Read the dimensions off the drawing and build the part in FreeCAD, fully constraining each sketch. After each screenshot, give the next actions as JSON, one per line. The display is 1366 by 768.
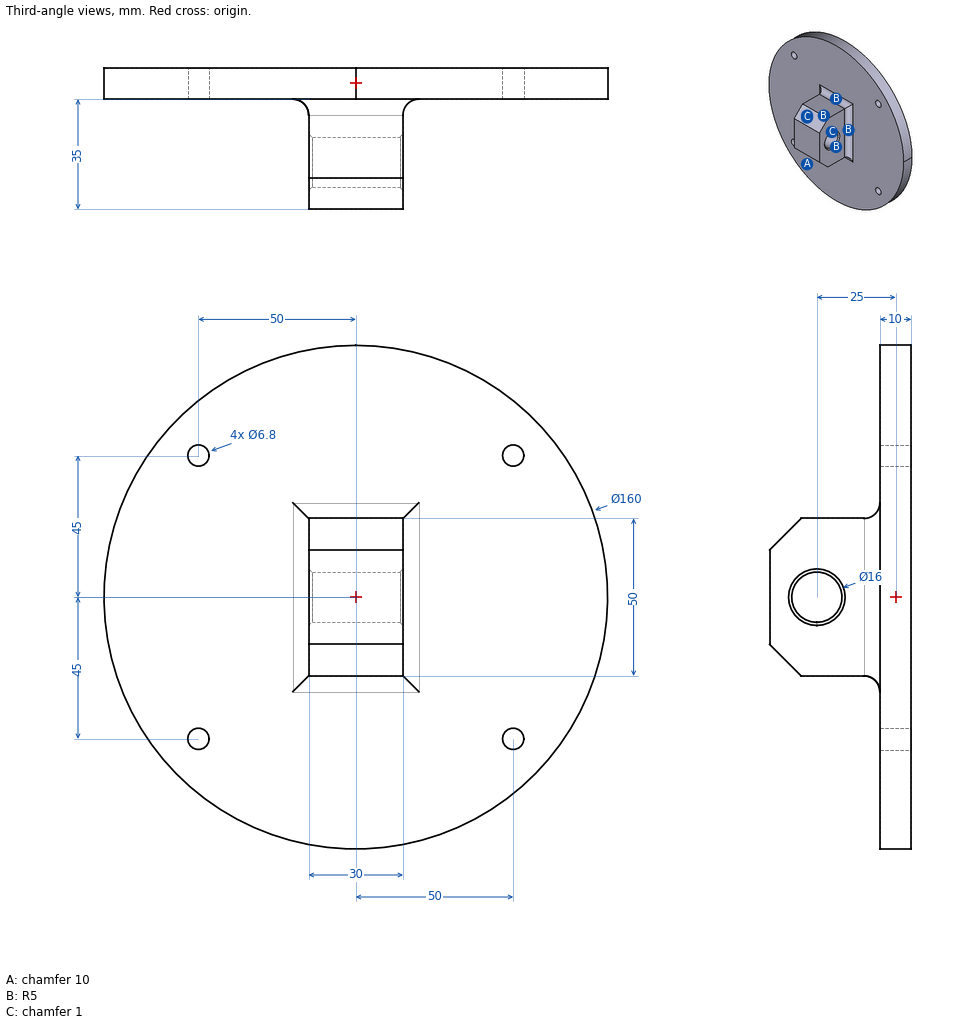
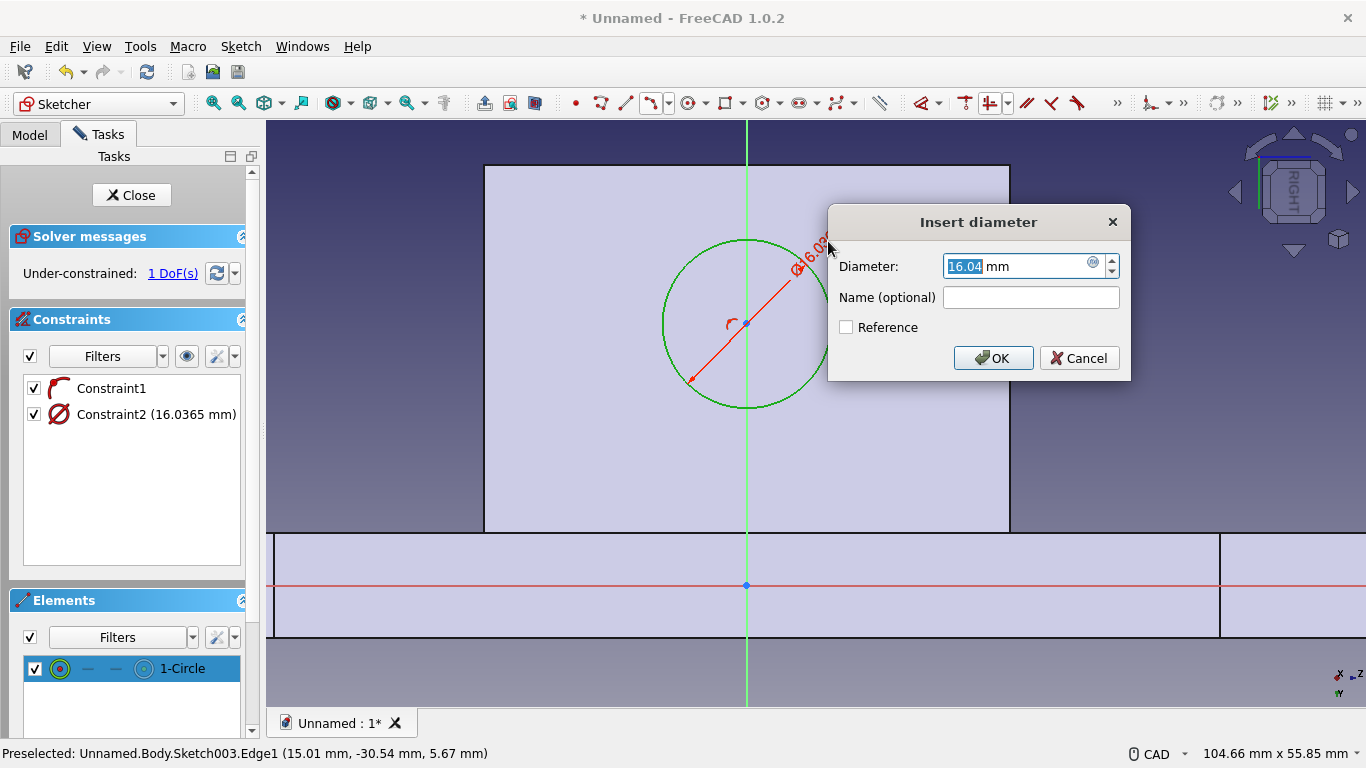
{"action": "type", "text": "16"}
{"action": "key", "text": "Return"}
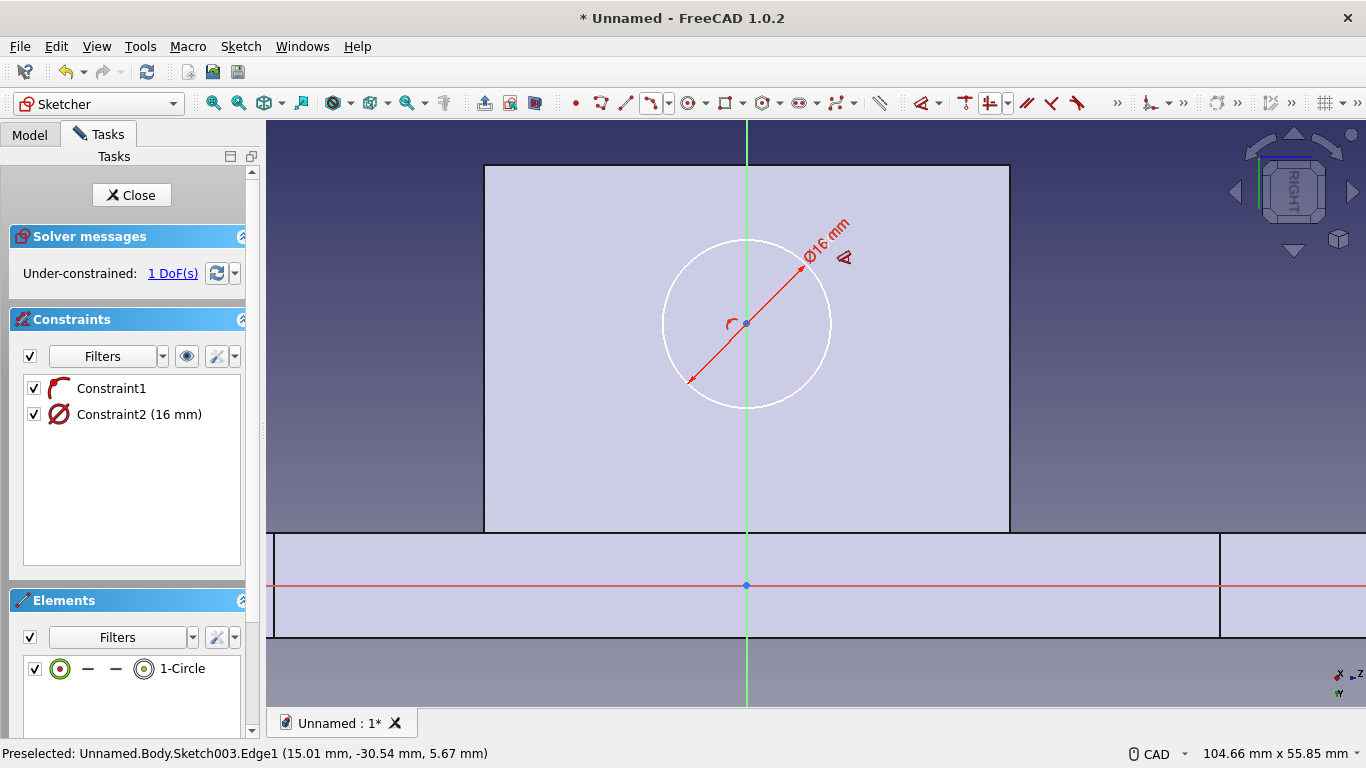
{"action": "left_click", "coordinate": [747, 324]}
{"action": "left_click", "coordinate": [781, 455]}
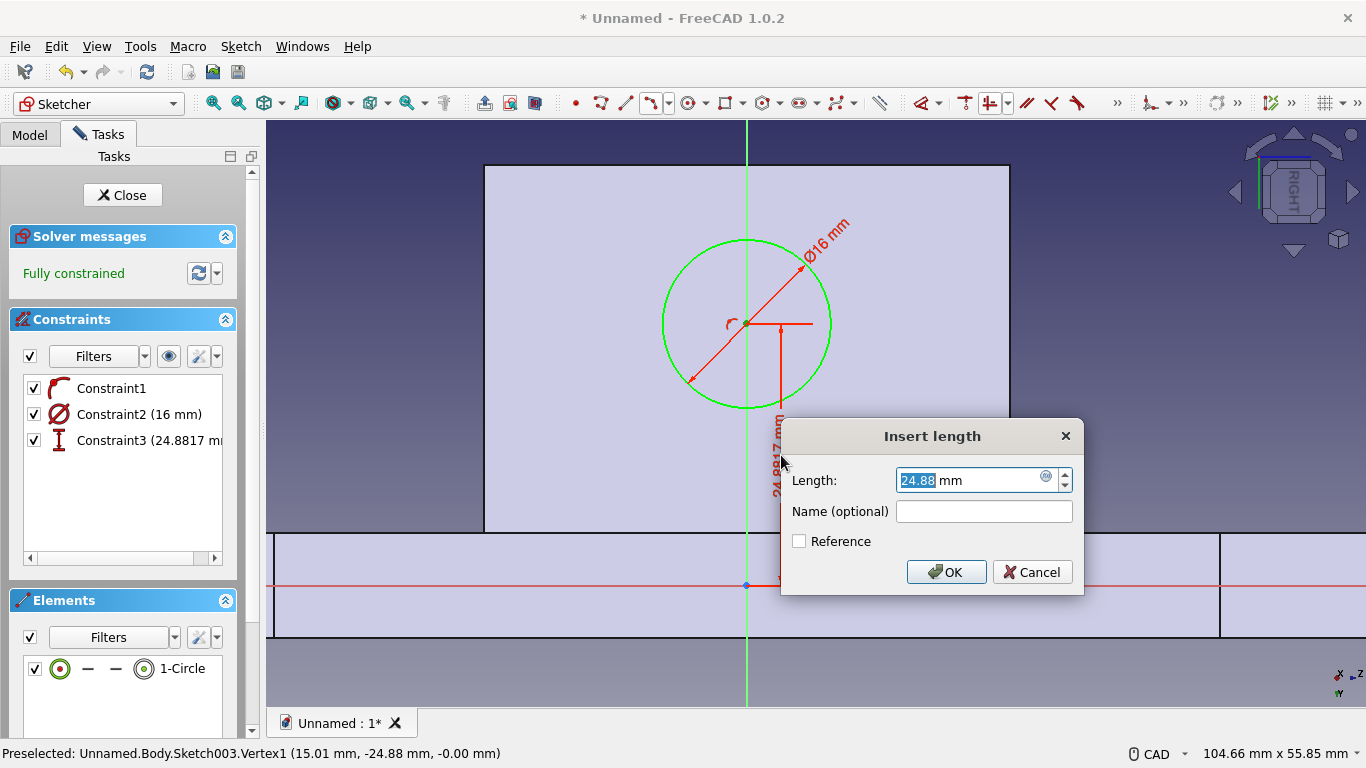
{"action": "type", "text": "25"}
{"action": "key", "text": "Return"}
{"action": "key", "text": "Escape"}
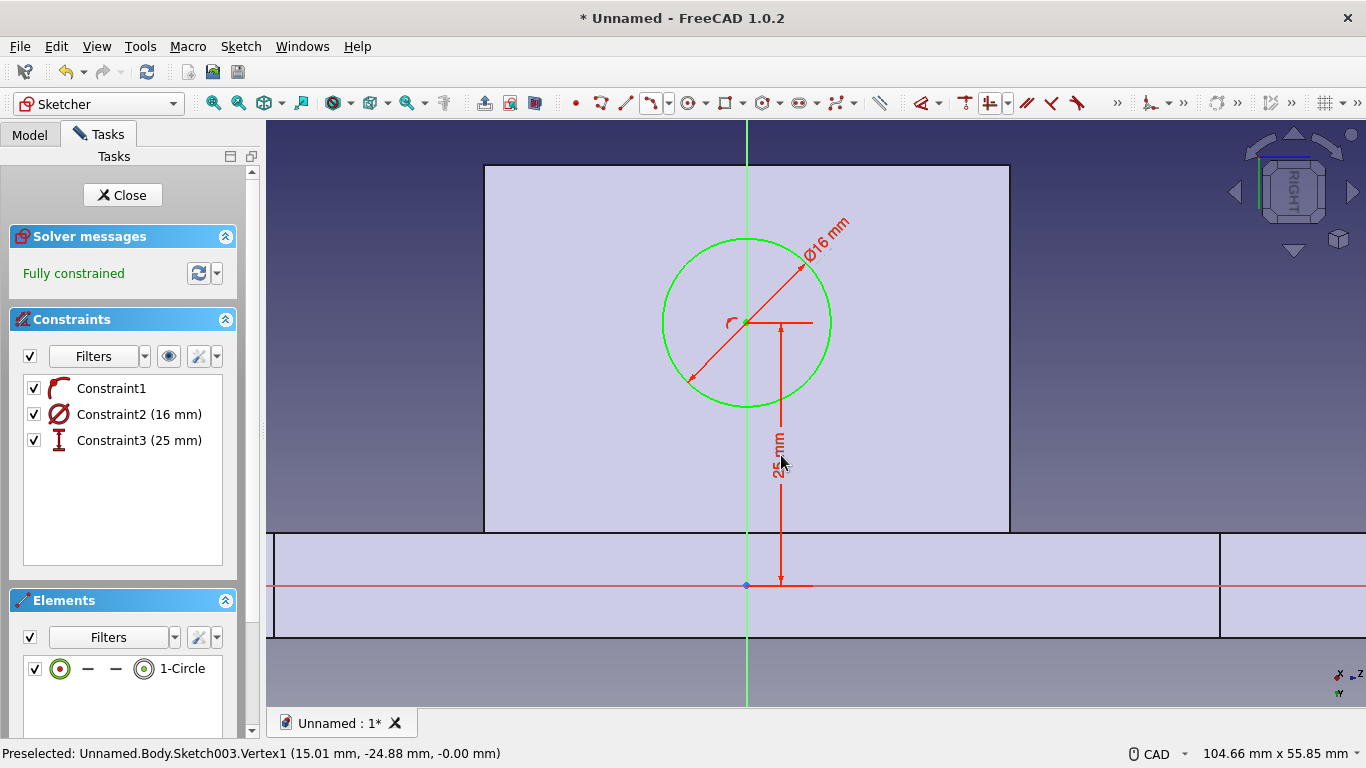
{"action": "left_click", "coordinate": [123, 195]}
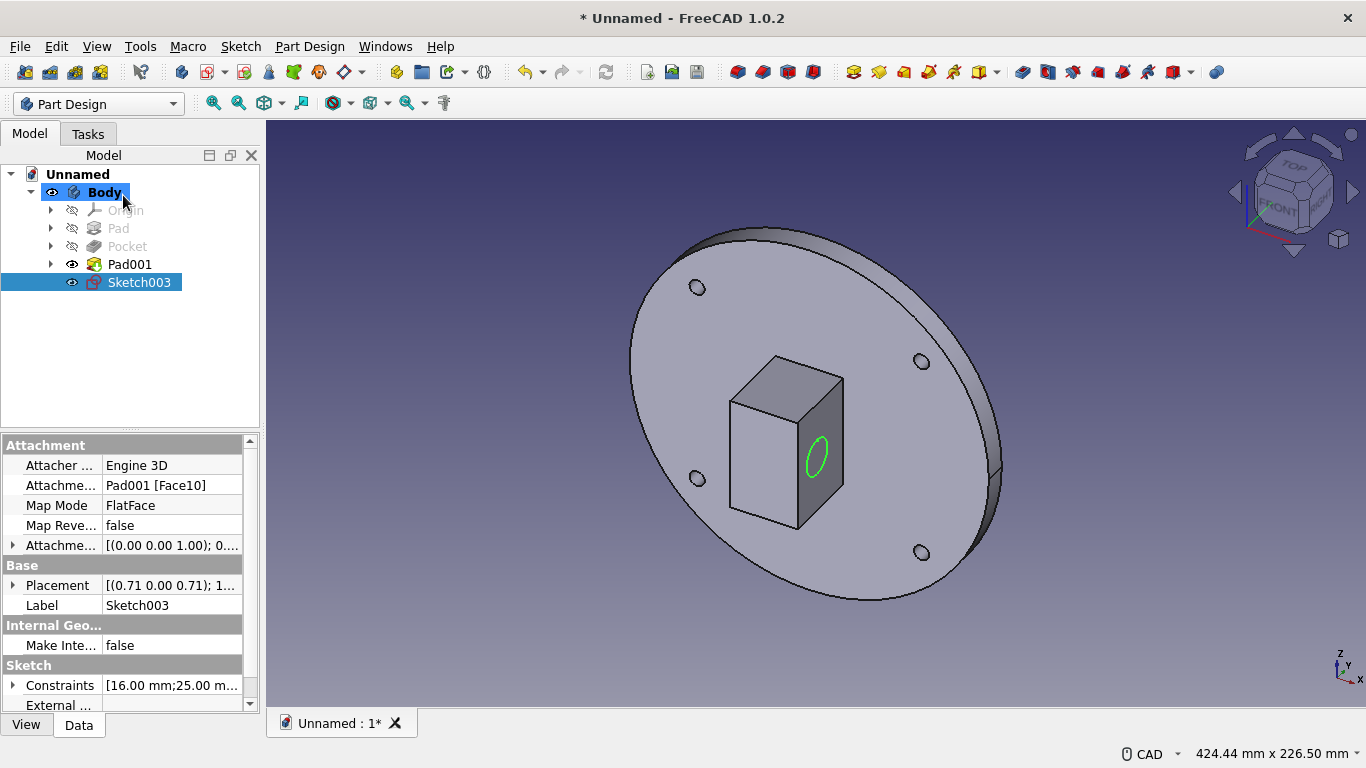
{"action": "left_click", "coordinate": [1023, 72]}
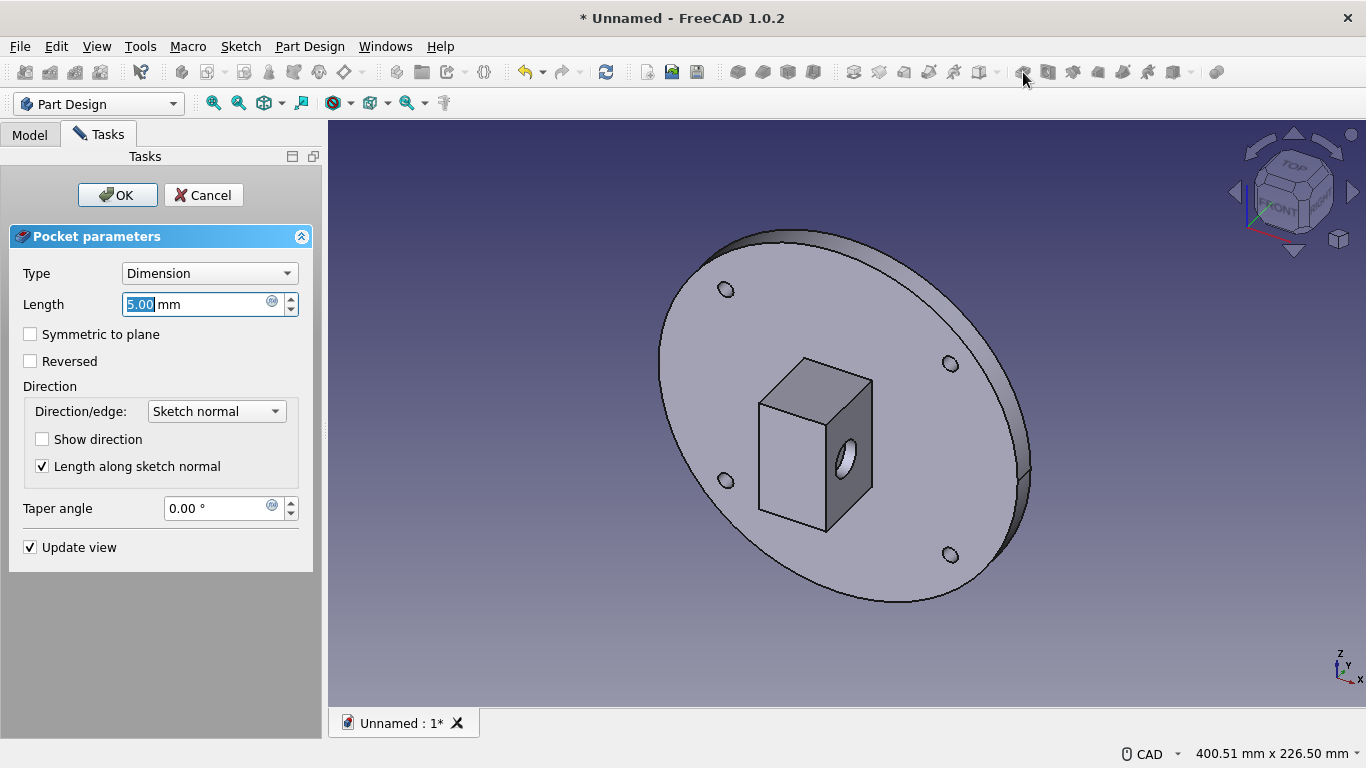
{"action": "left_click", "coordinate": [210, 274]}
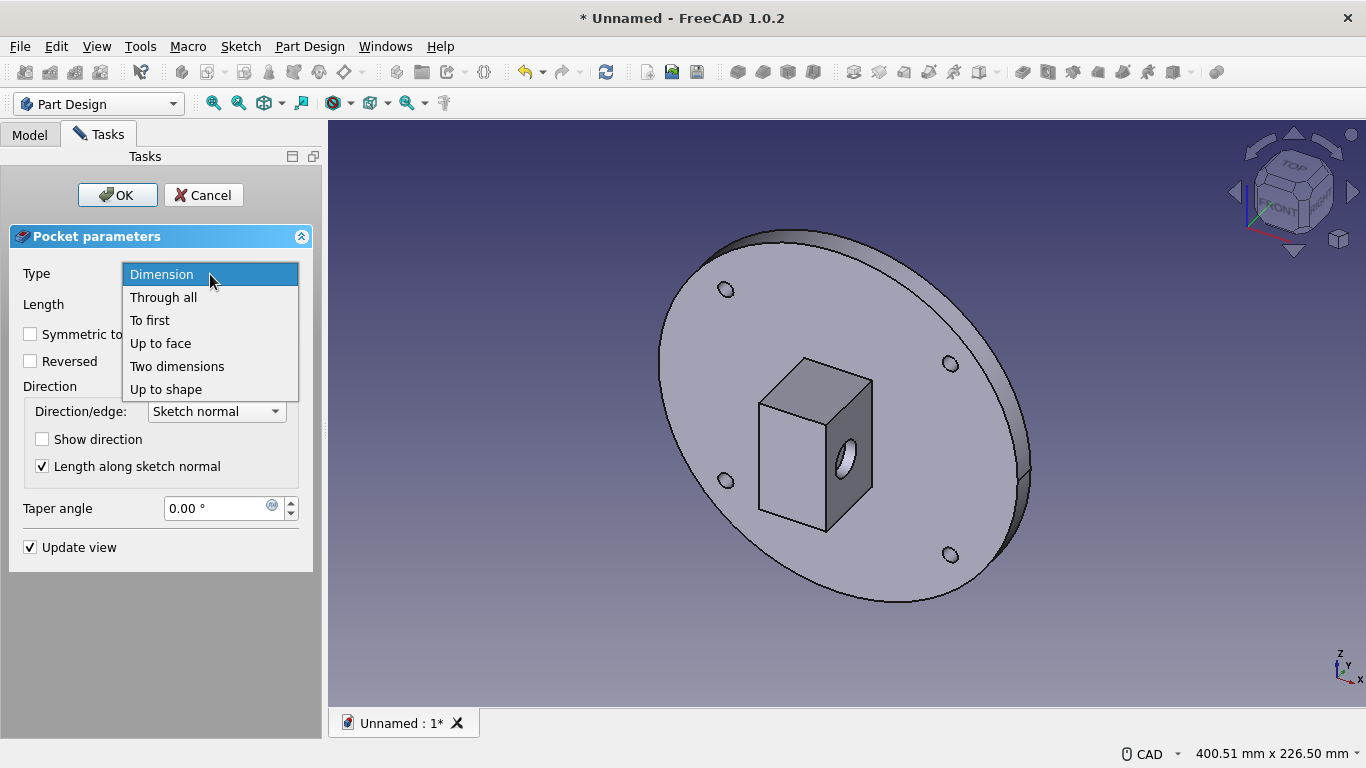
{"action": "left_click", "coordinate": [208, 298]}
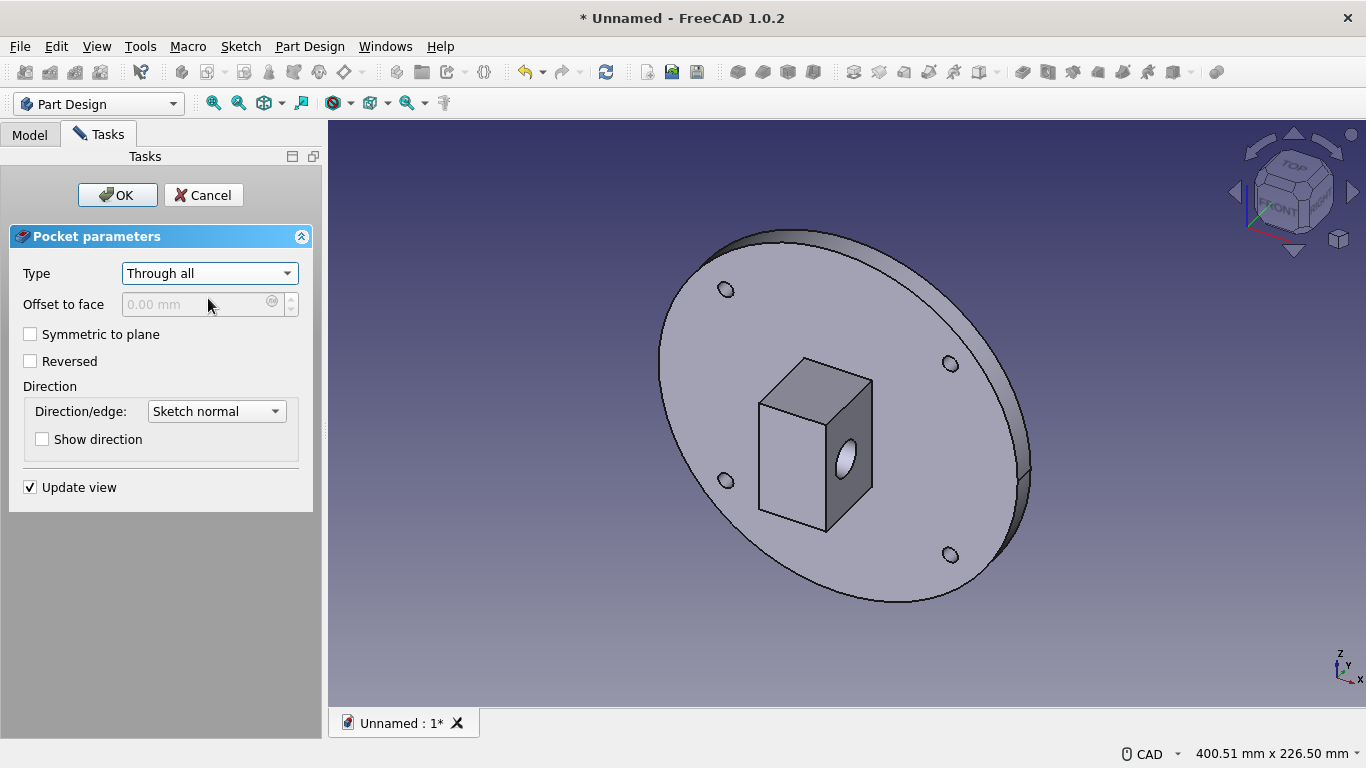
{"action": "left_click", "coordinate": [118, 195]}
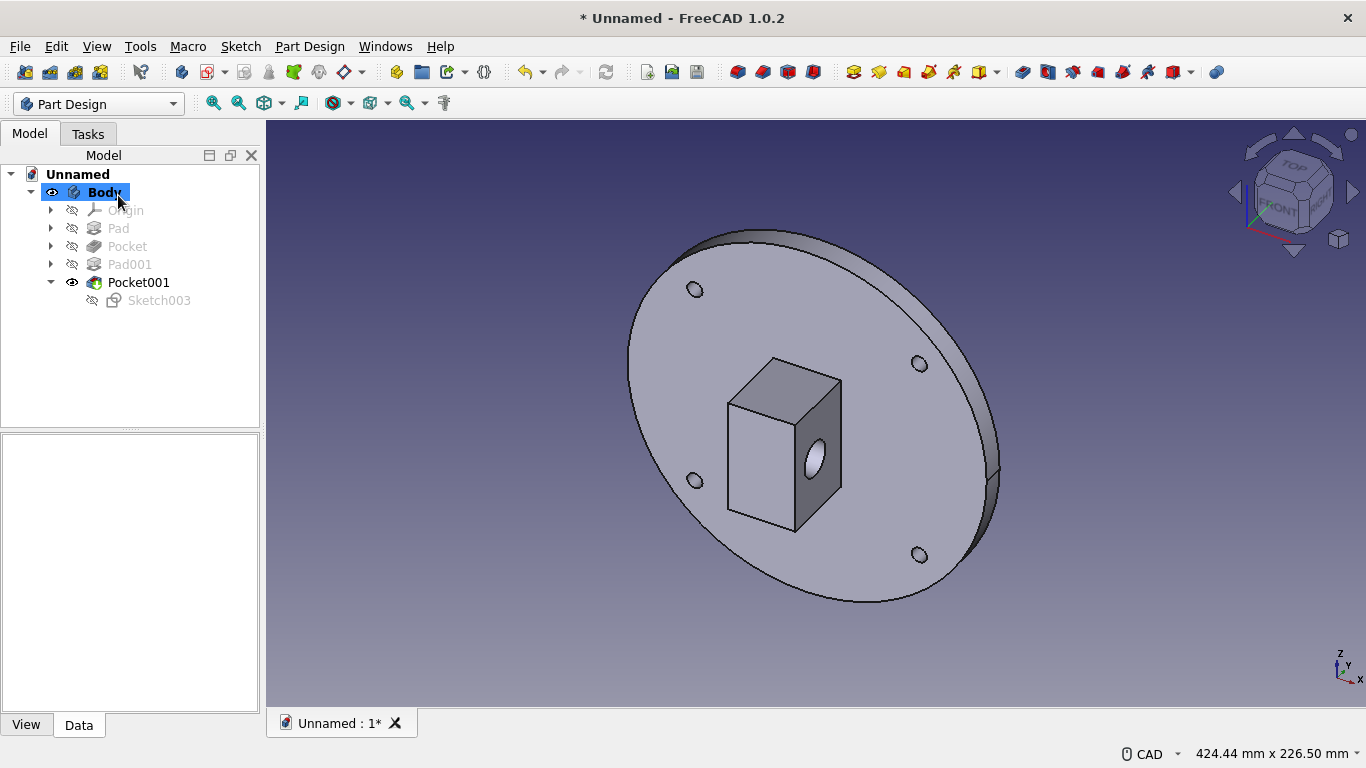
{"action": "left_click", "coordinate": [762, 413]}